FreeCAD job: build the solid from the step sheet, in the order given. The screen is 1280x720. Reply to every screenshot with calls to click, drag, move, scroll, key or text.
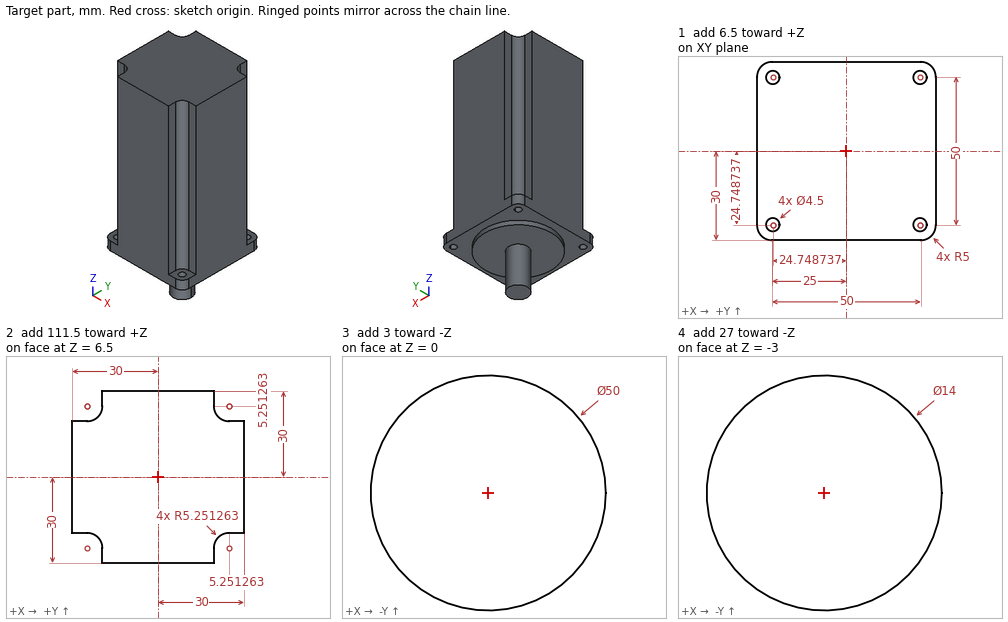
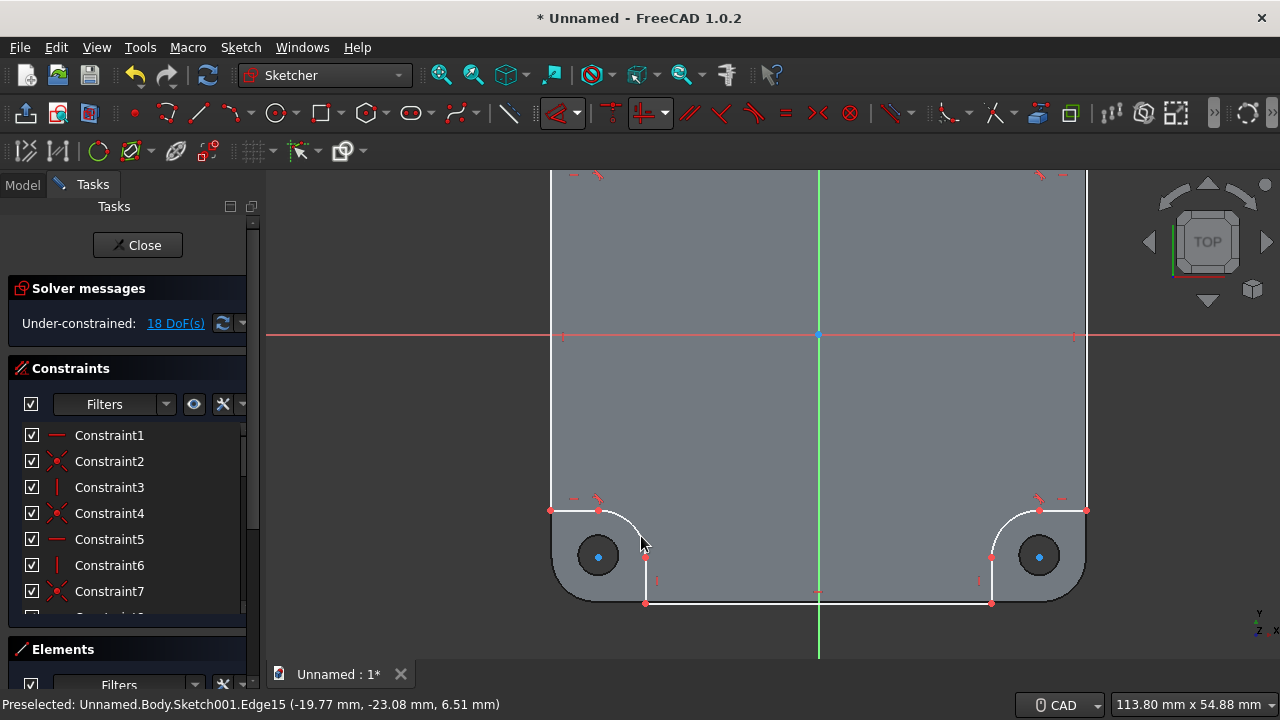
click(646, 572)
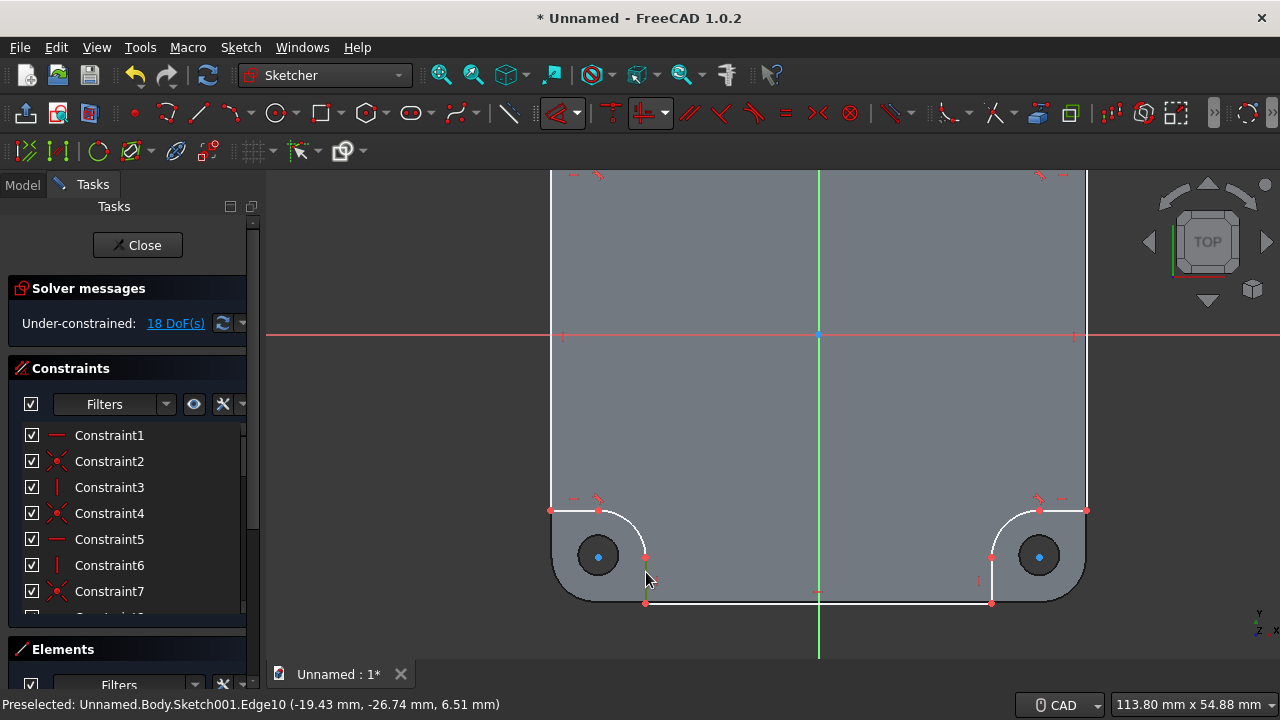
click(641, 536)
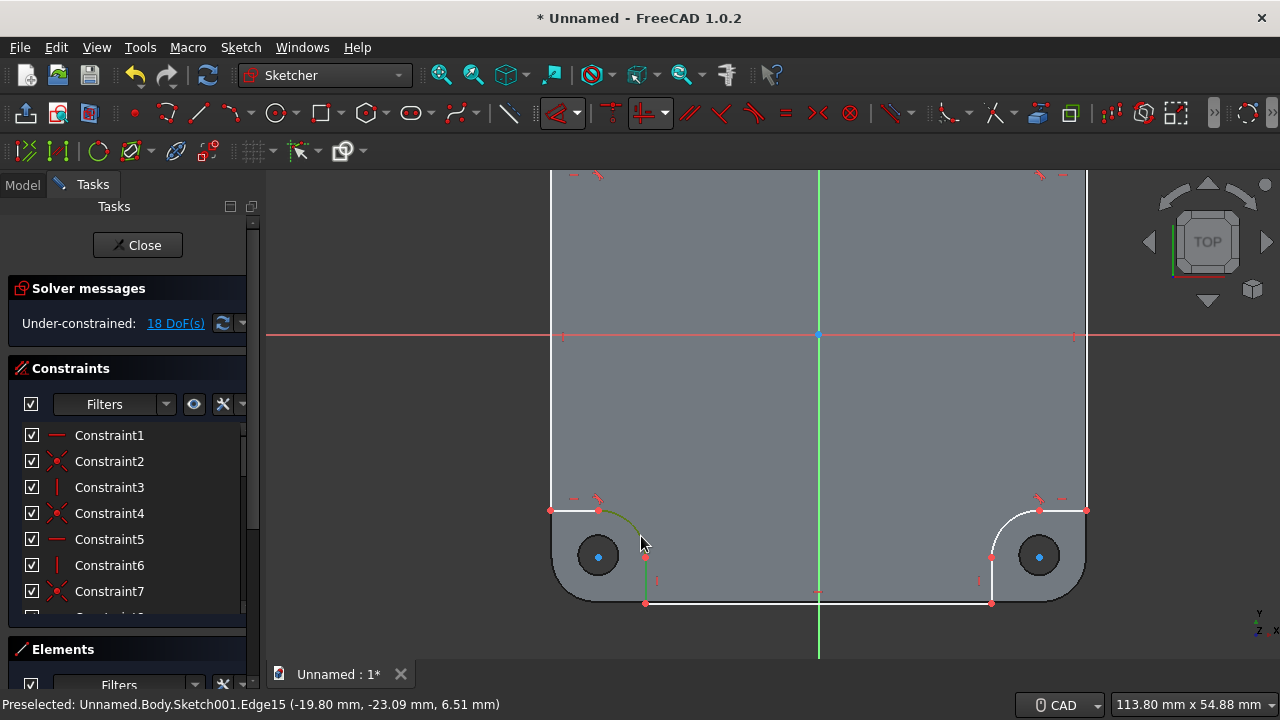
key(t)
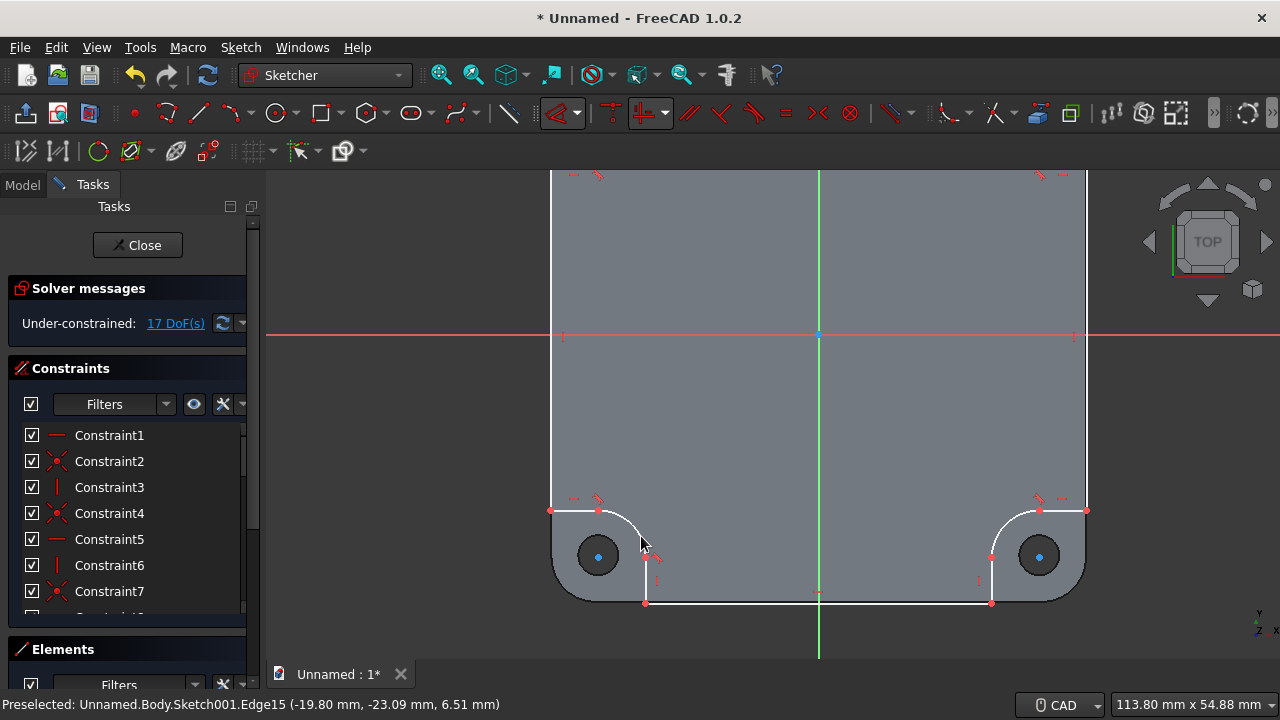
click(992, 590)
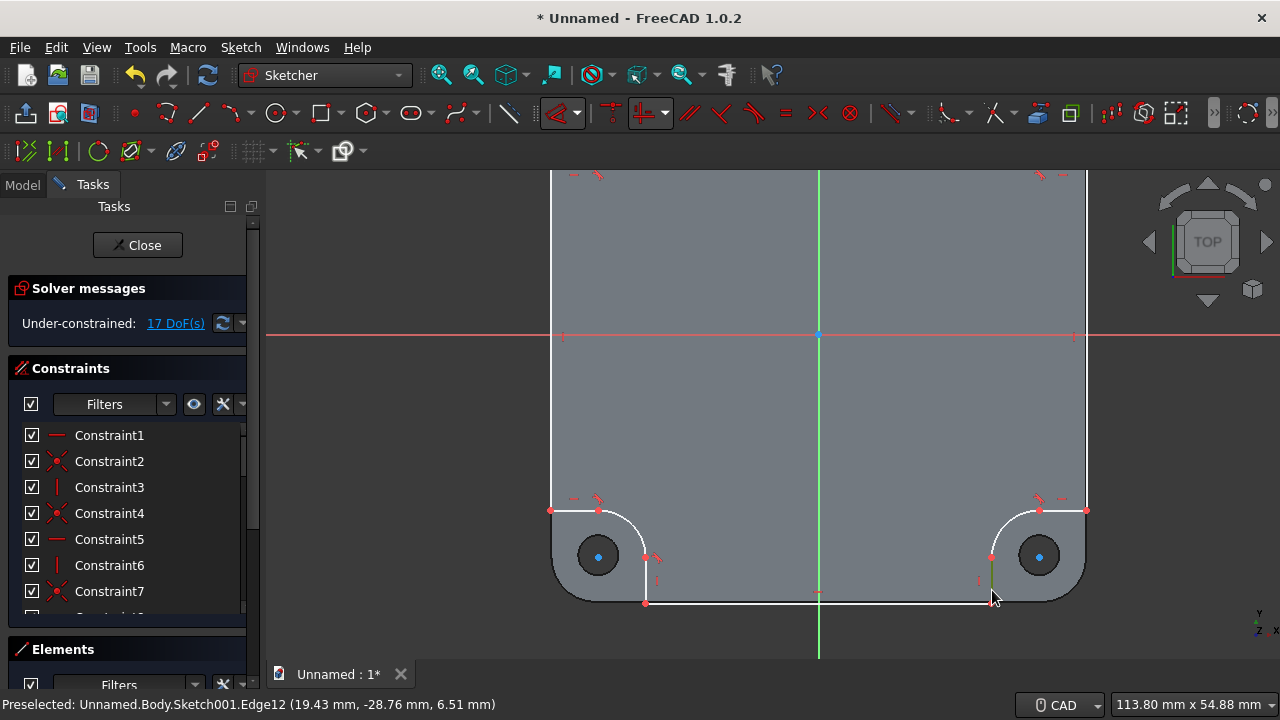
click(1018, 516)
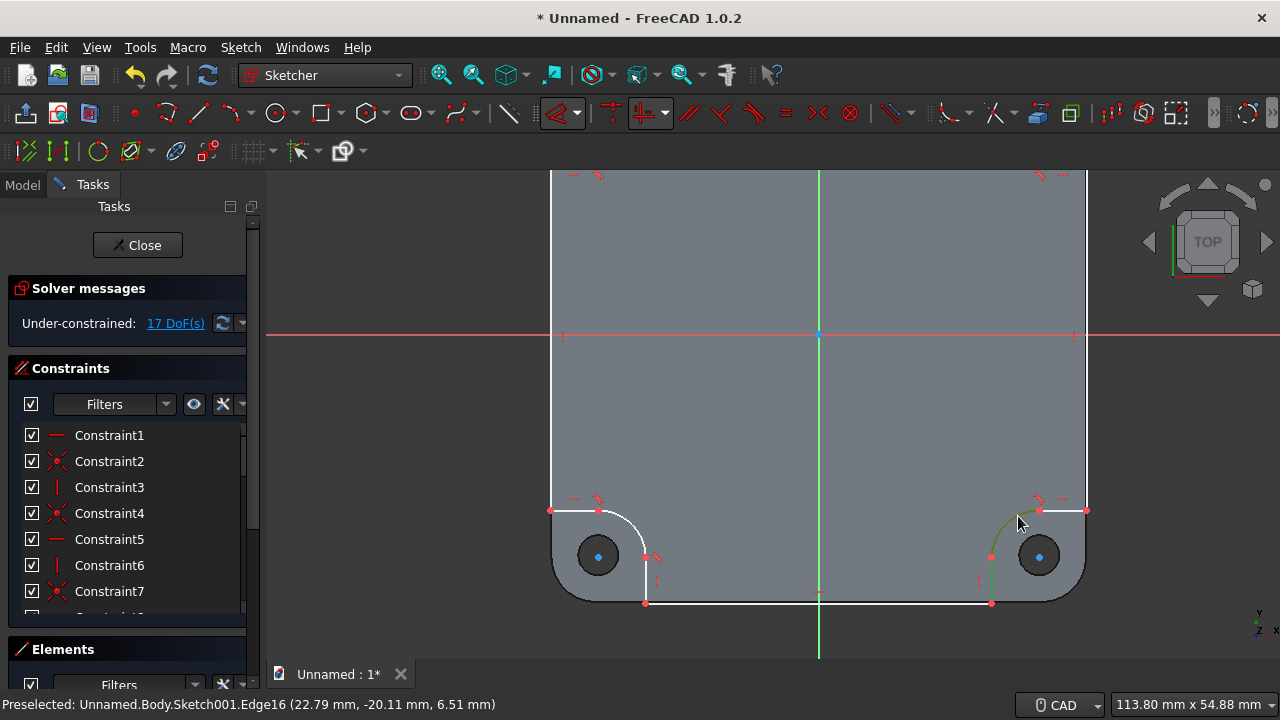
key(t)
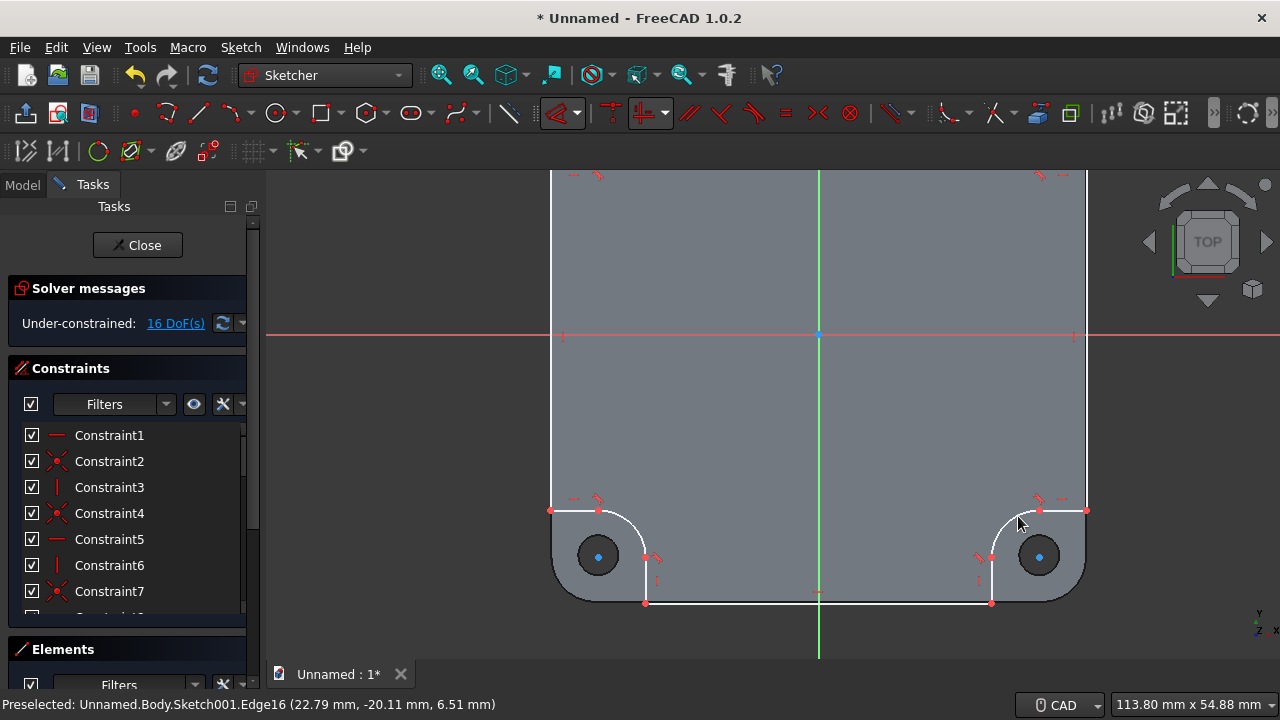
scroll(565, 511, down, 3)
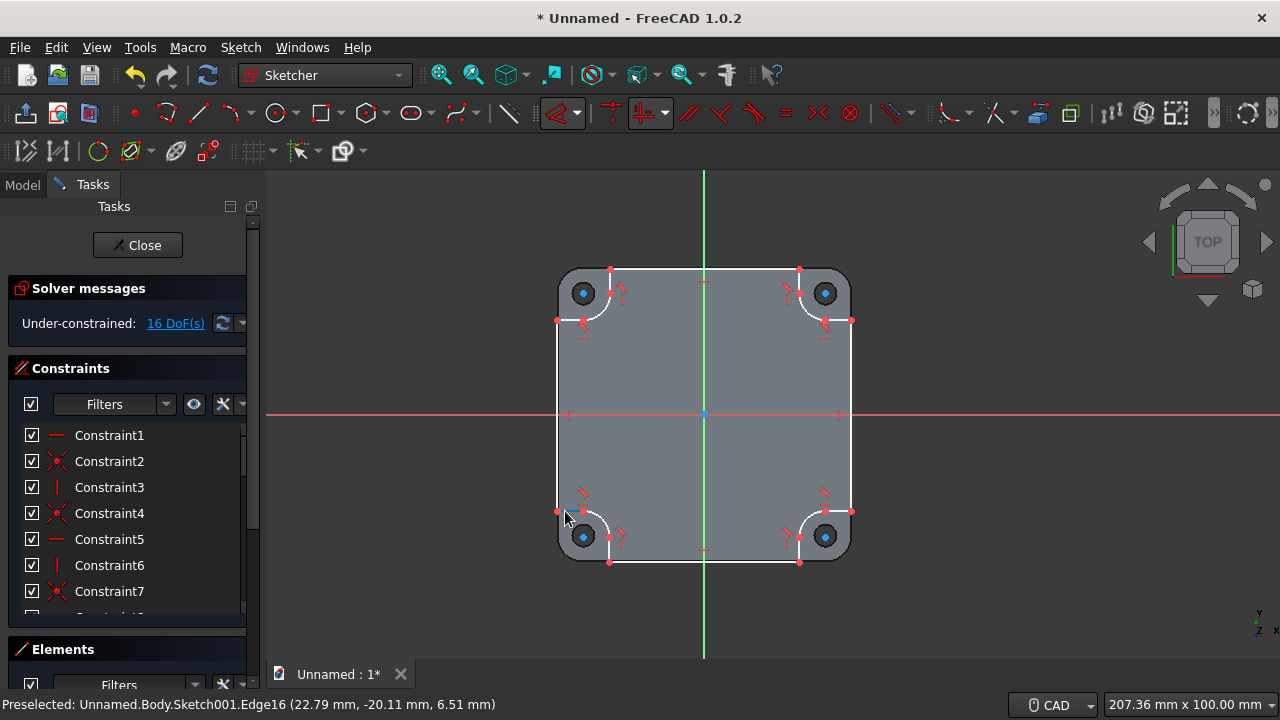
click(802, 306)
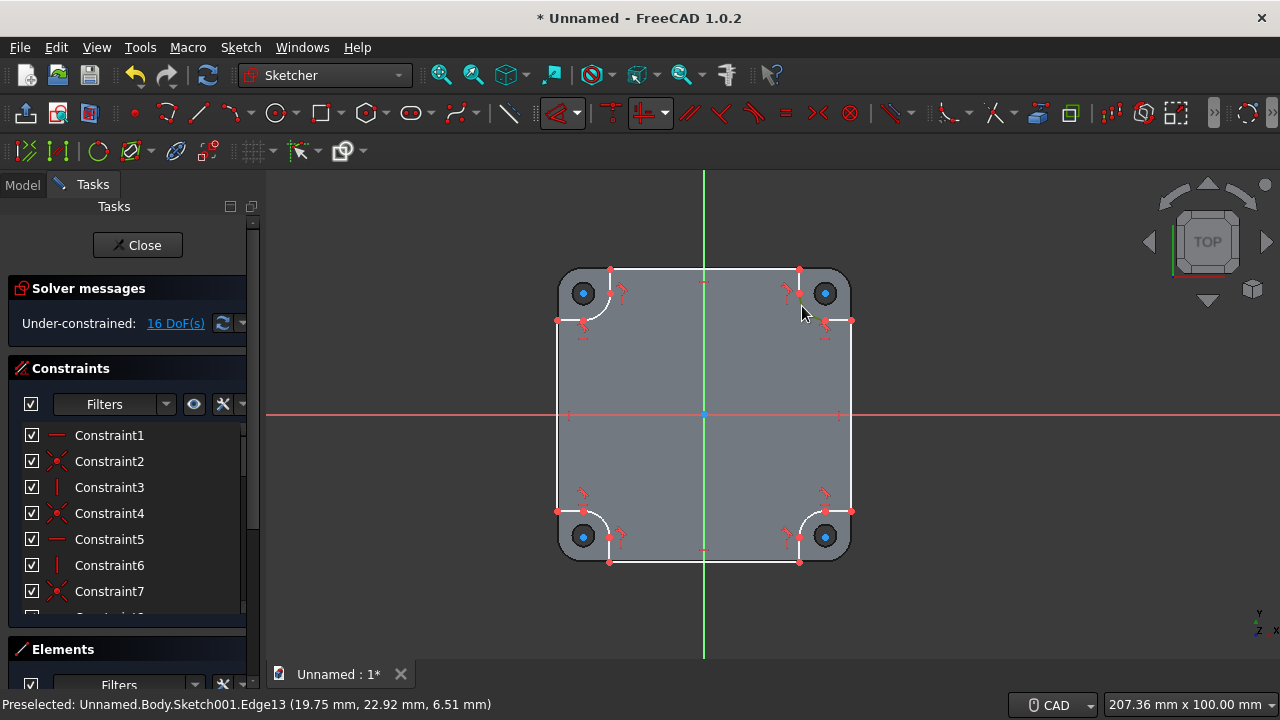
click(596, 317)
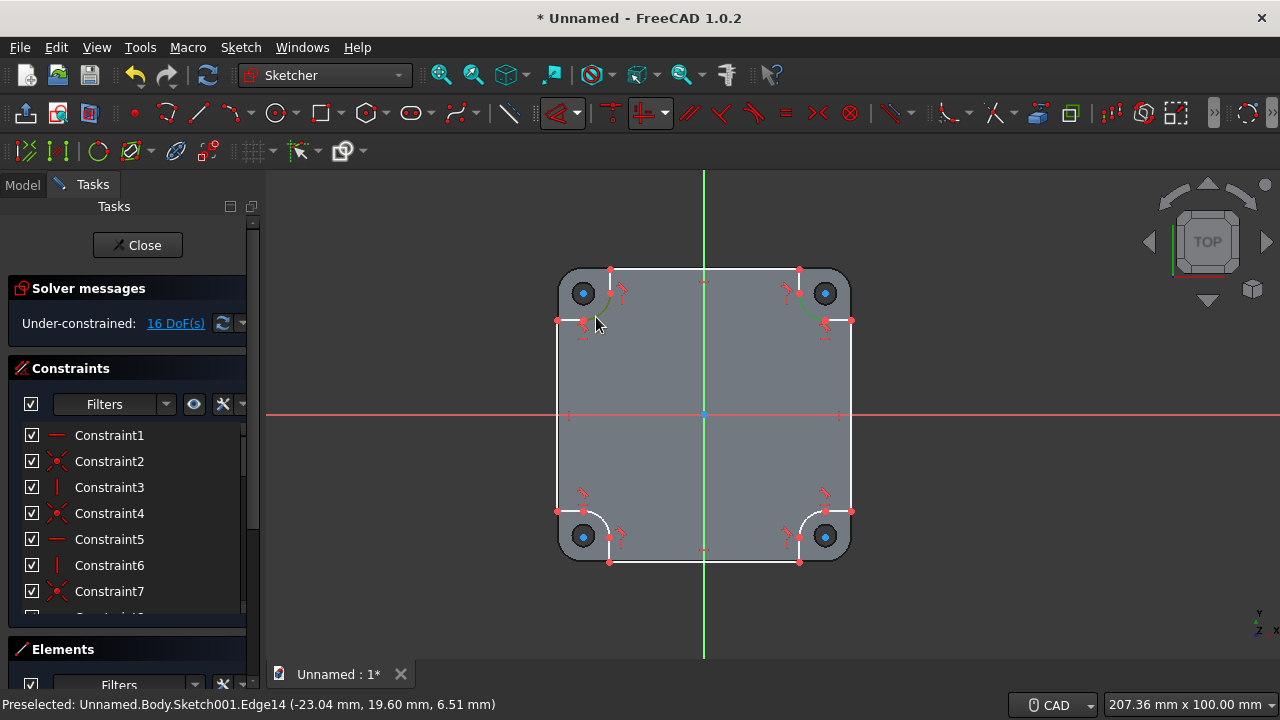
click(607, 525)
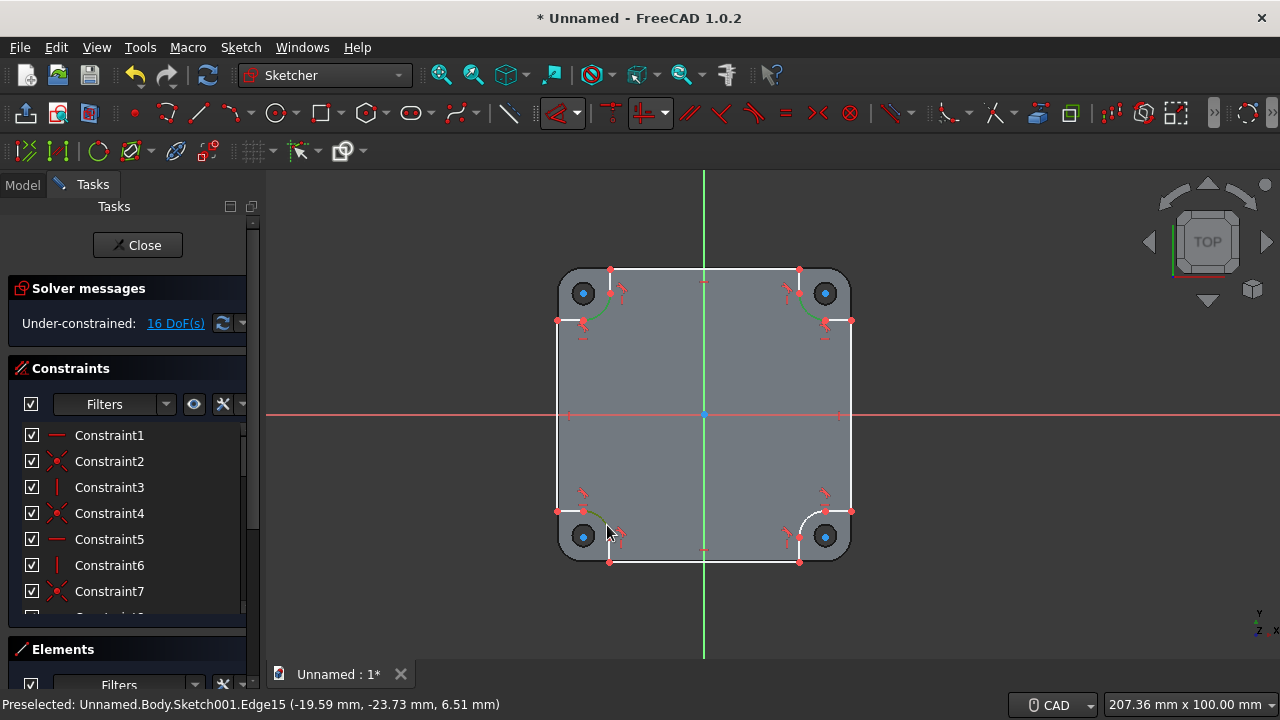
click(814, 514)